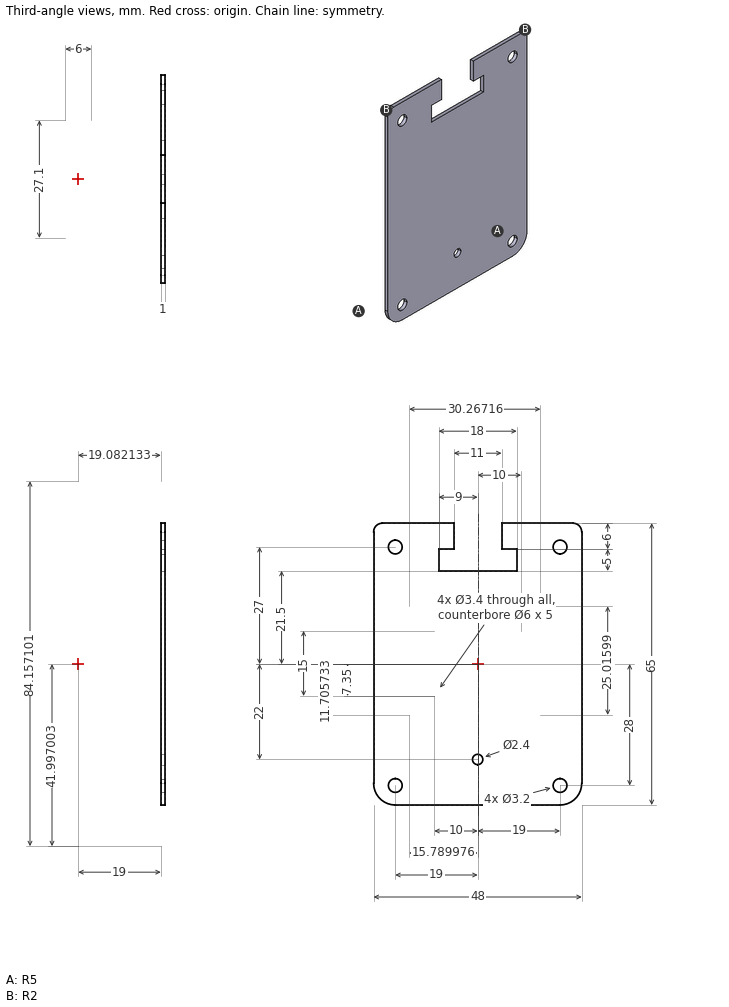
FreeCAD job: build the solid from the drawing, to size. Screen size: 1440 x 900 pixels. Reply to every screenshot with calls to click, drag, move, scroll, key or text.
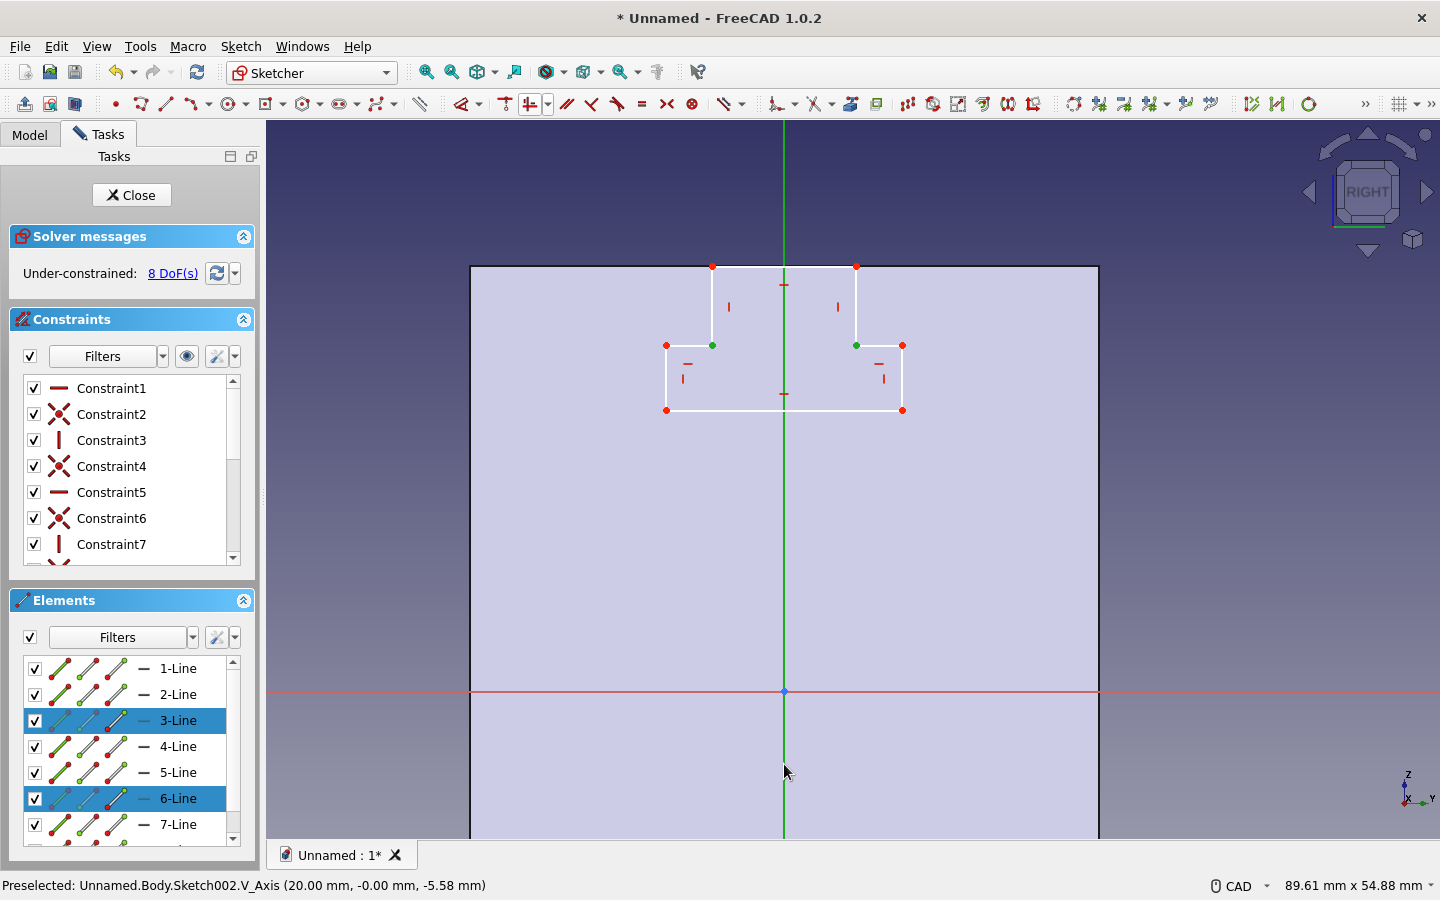
key(s)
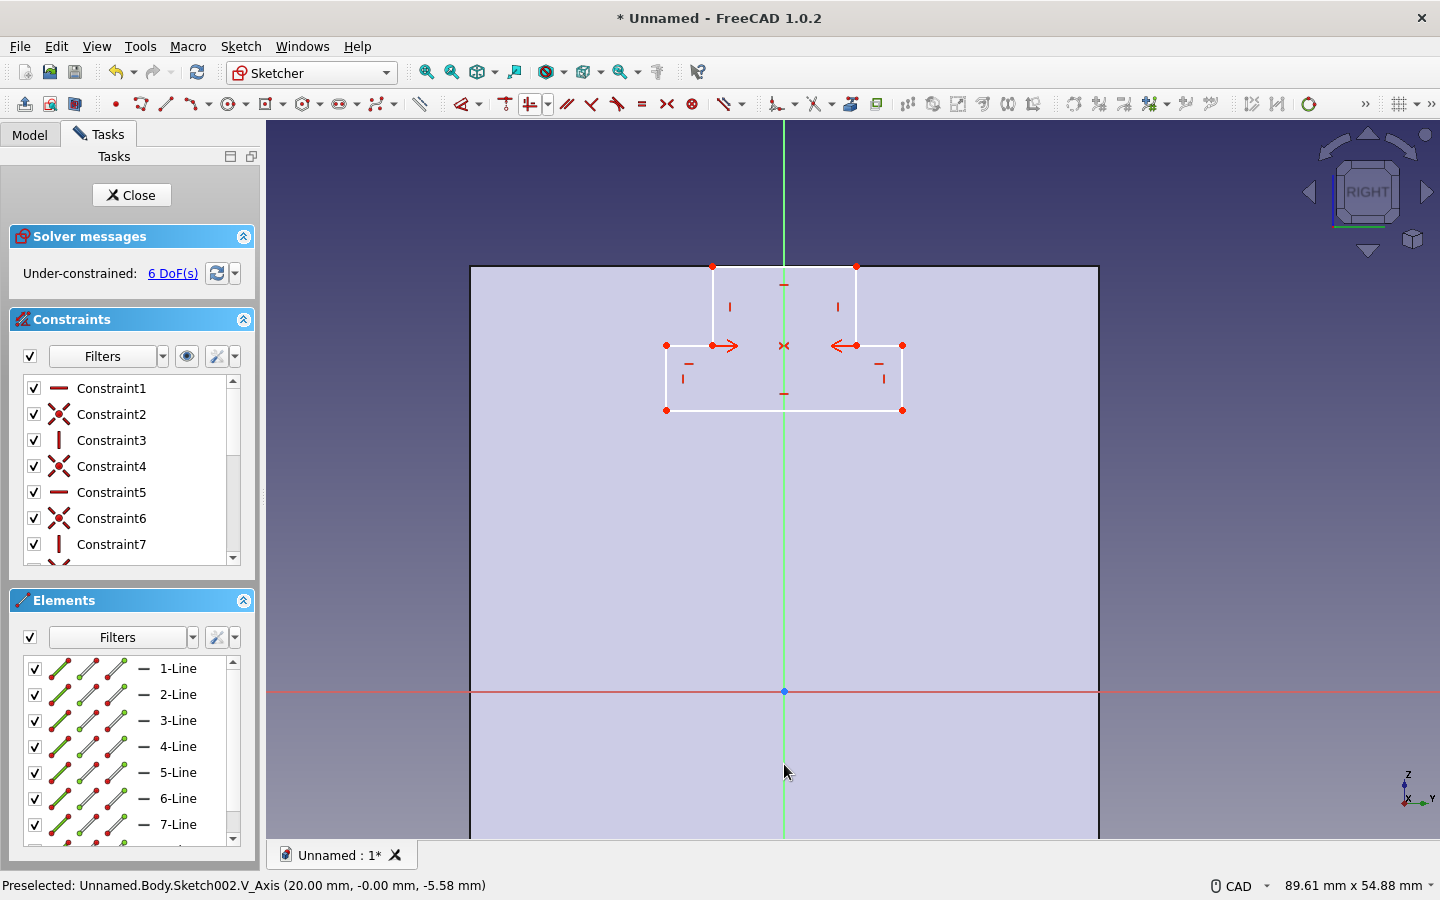
click(902, 391)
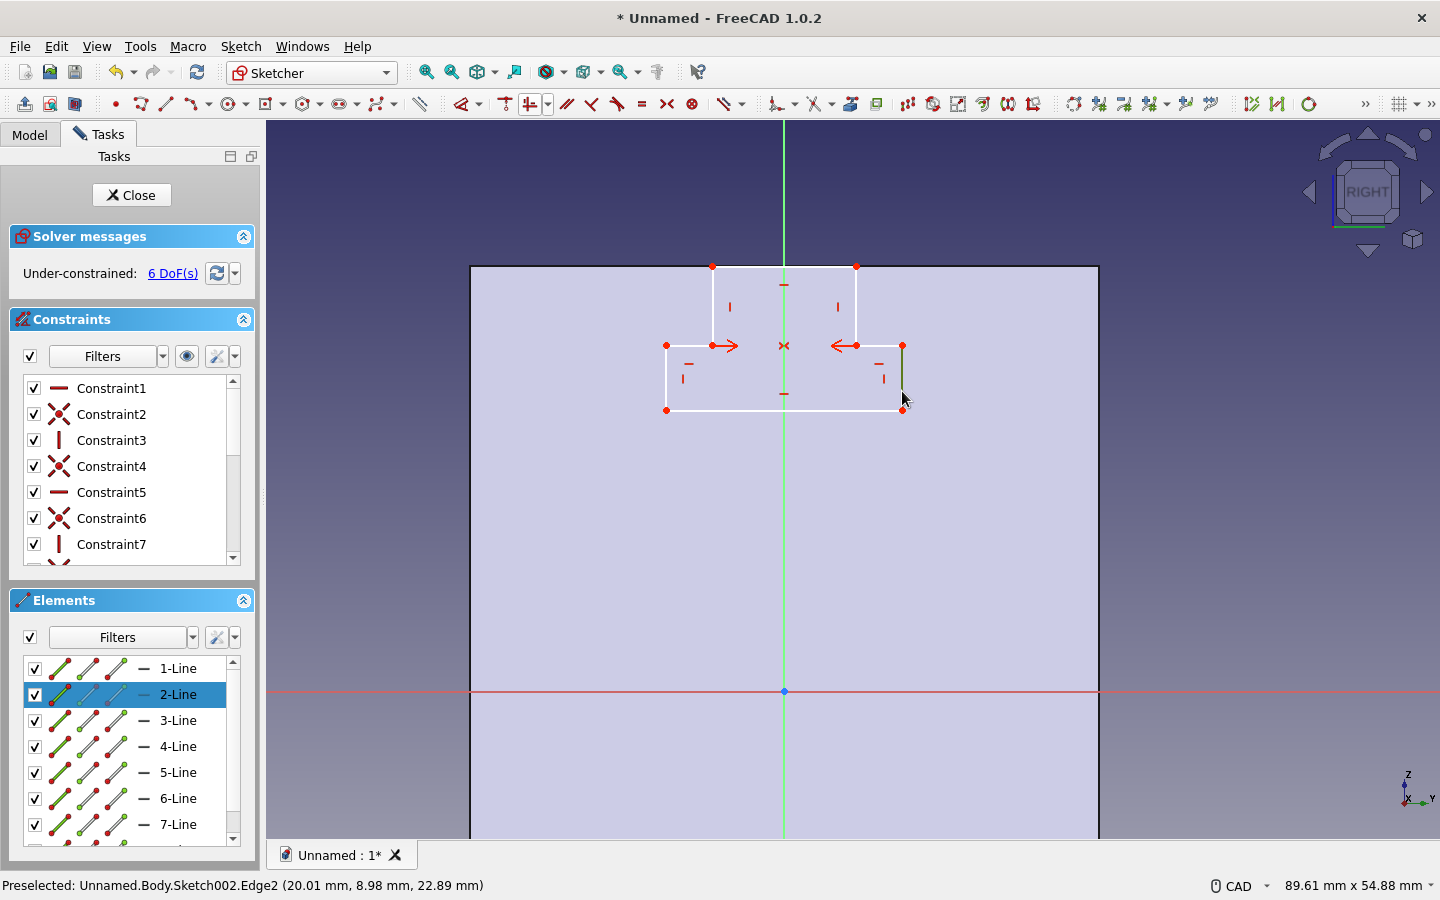
key(i)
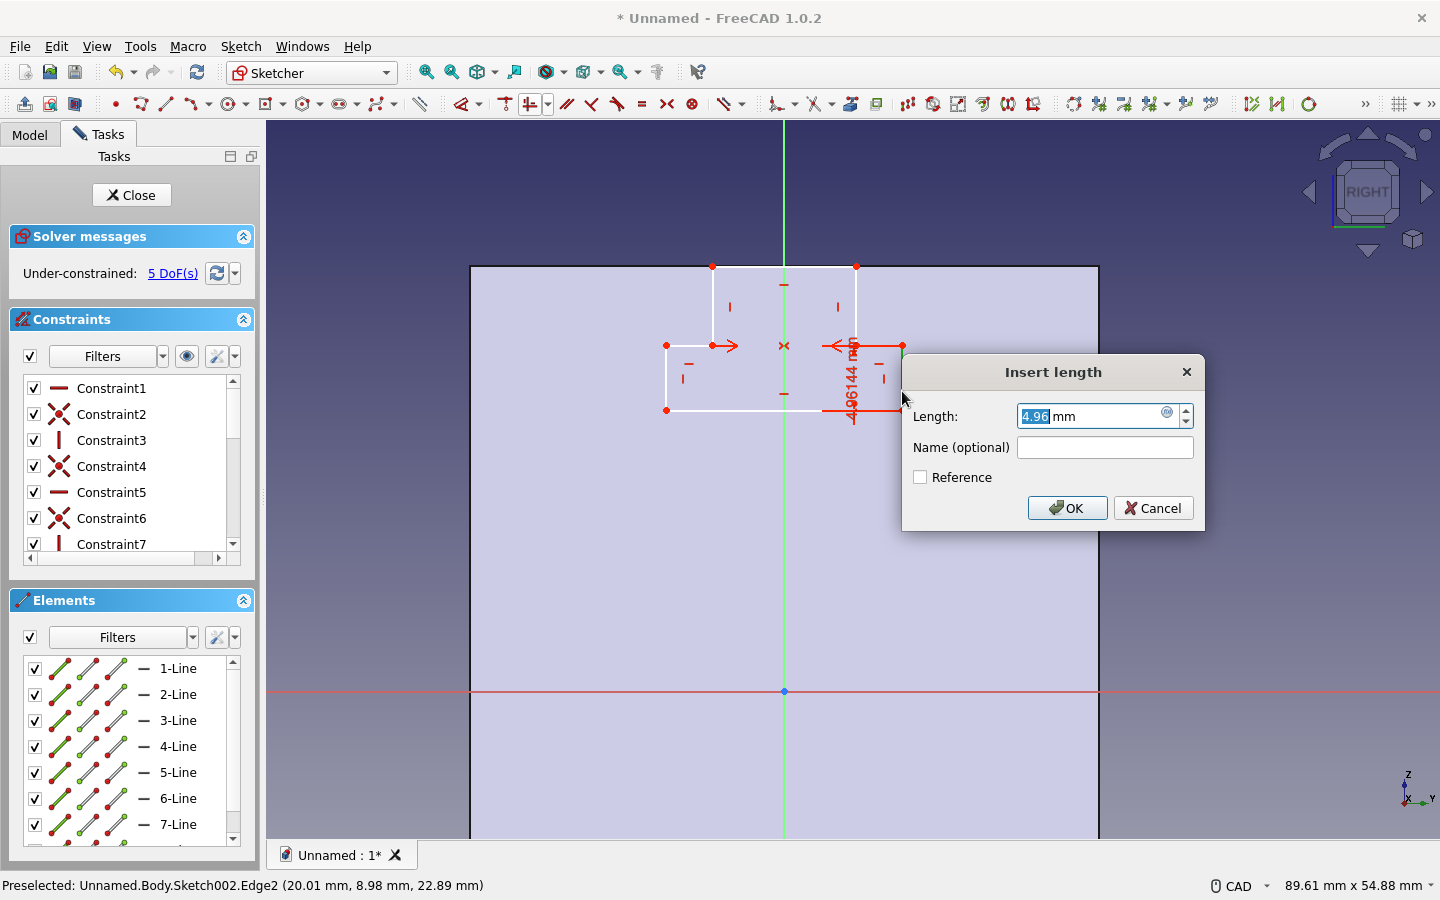
text(5)
key(Return)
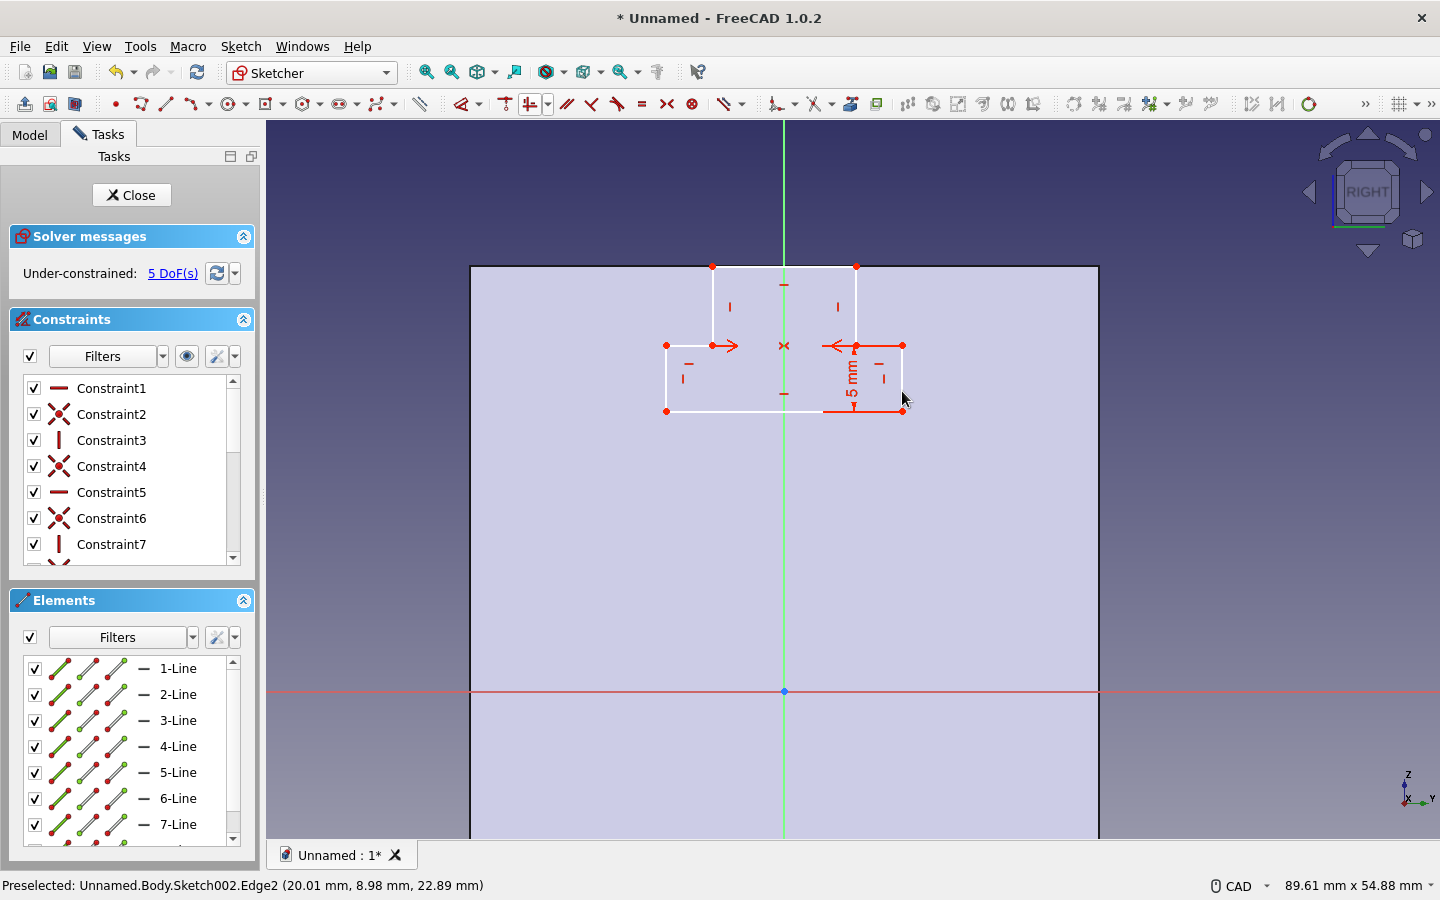
click(856, 322)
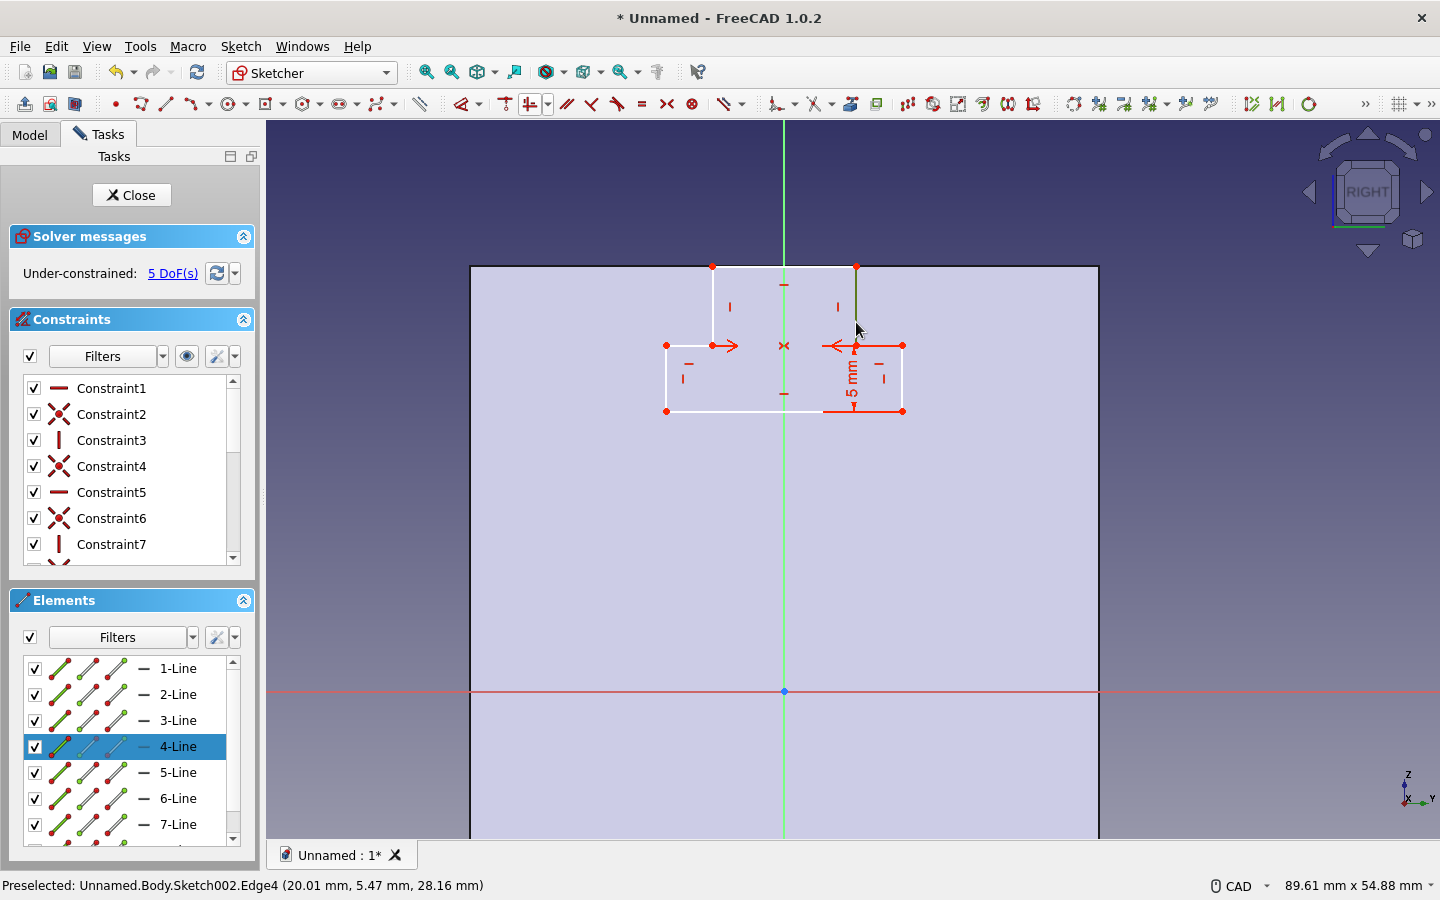
key(i)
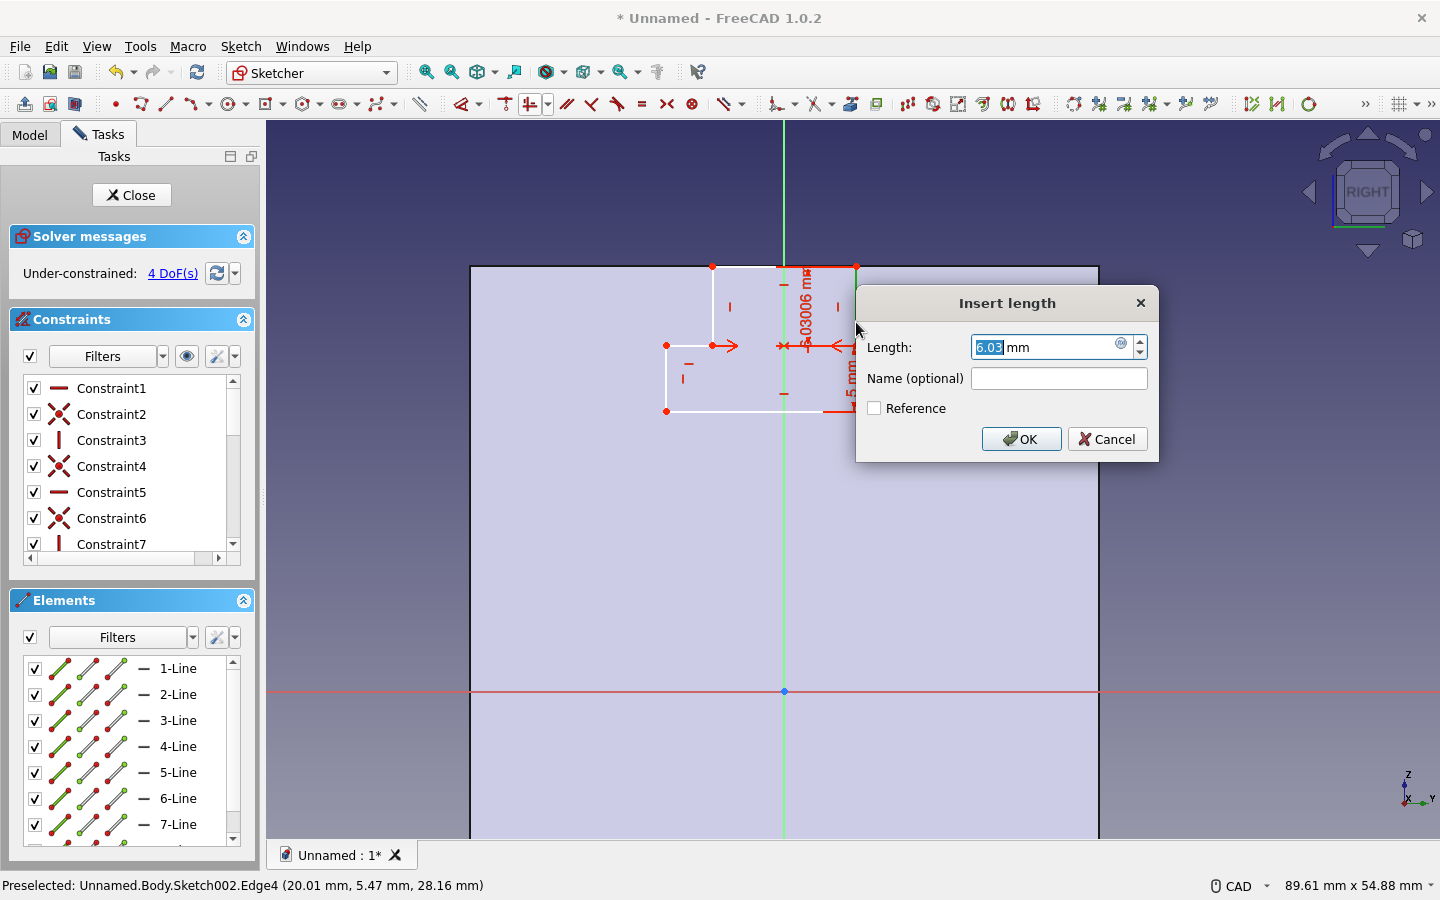
text(6)
key(Return)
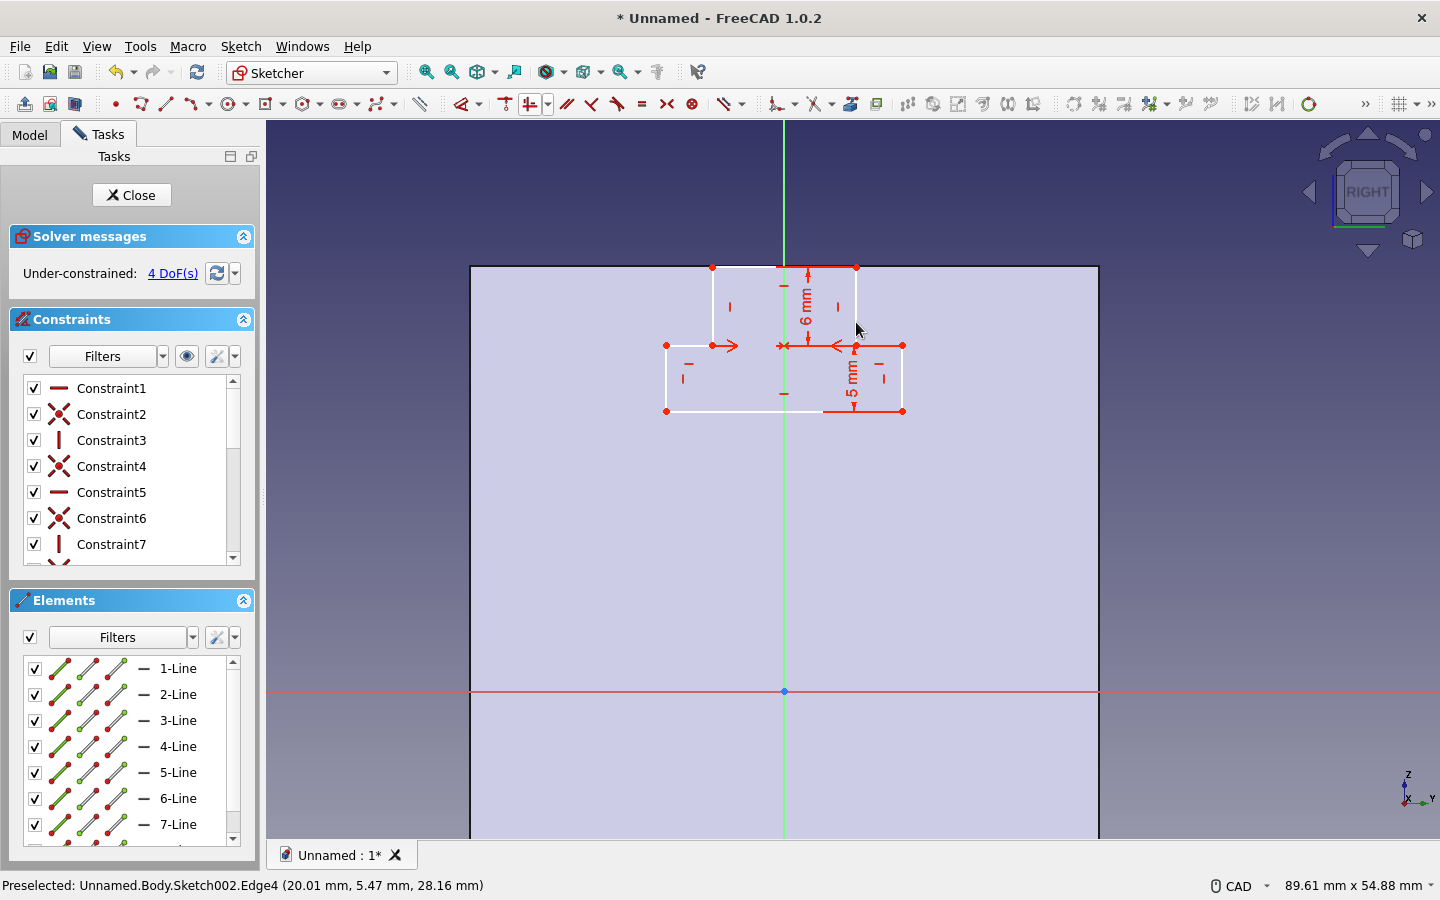
click(737, 412)